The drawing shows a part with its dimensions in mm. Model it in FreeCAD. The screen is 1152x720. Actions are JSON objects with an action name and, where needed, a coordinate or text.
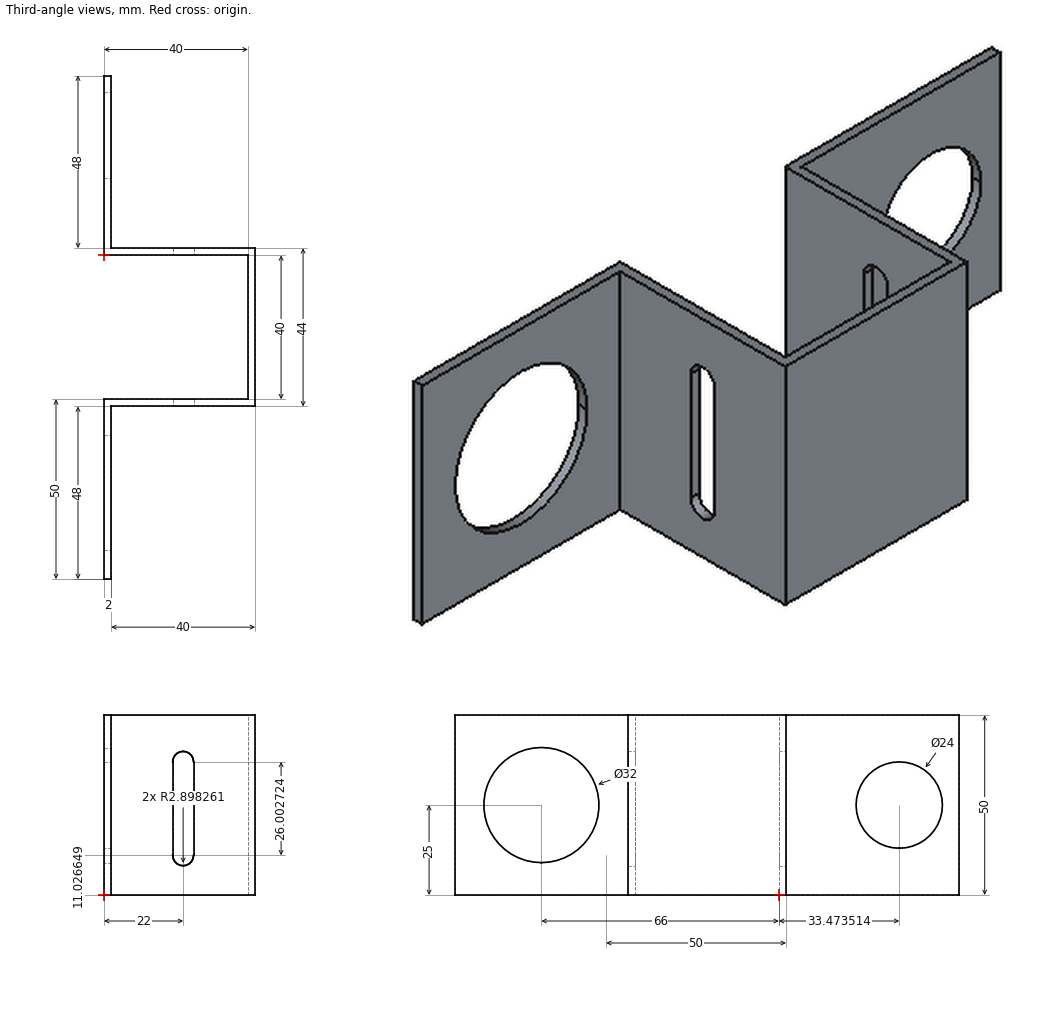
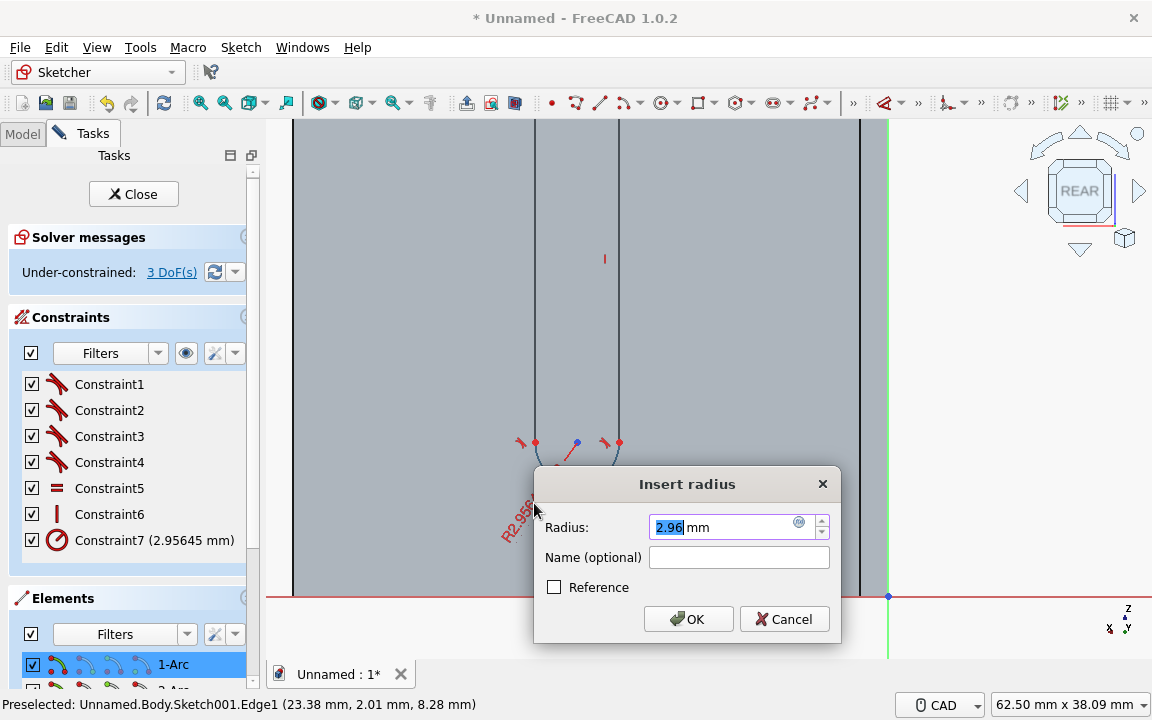
{"action": "type", "text": "2.898261"}
{"action": "key", "text": "Return"}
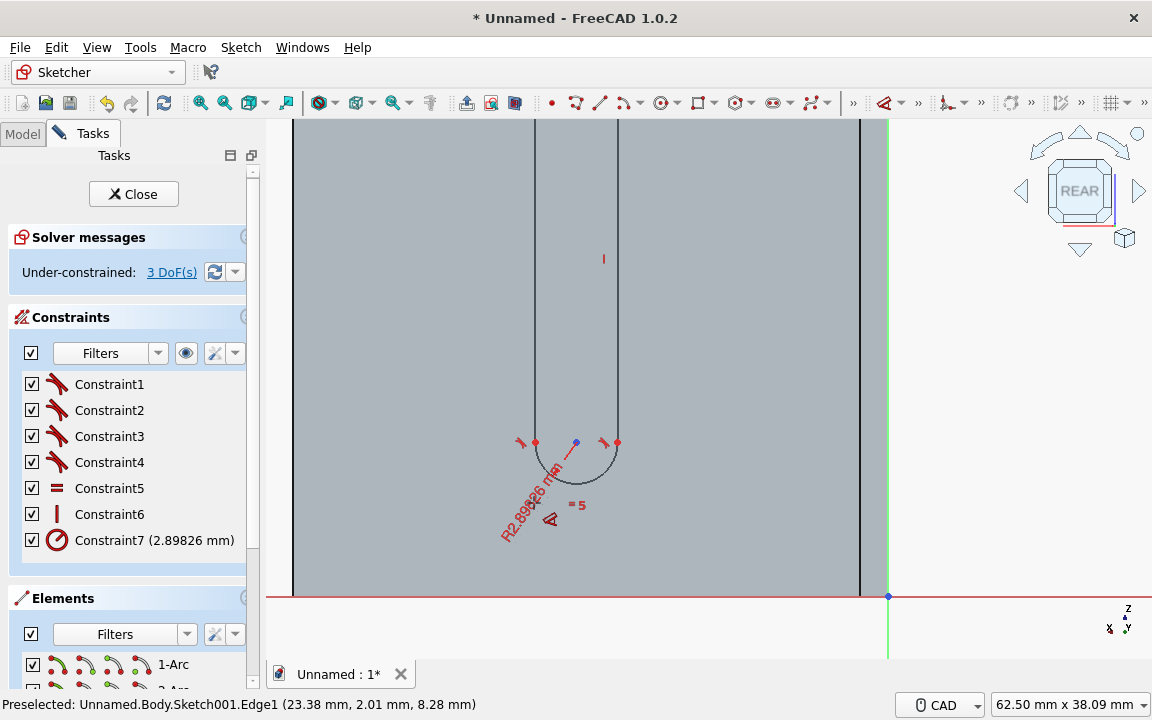
{"action": "left_click", "coordinate": [576, 443]}
{"action": "left_click", "coordinate": [732, 631]}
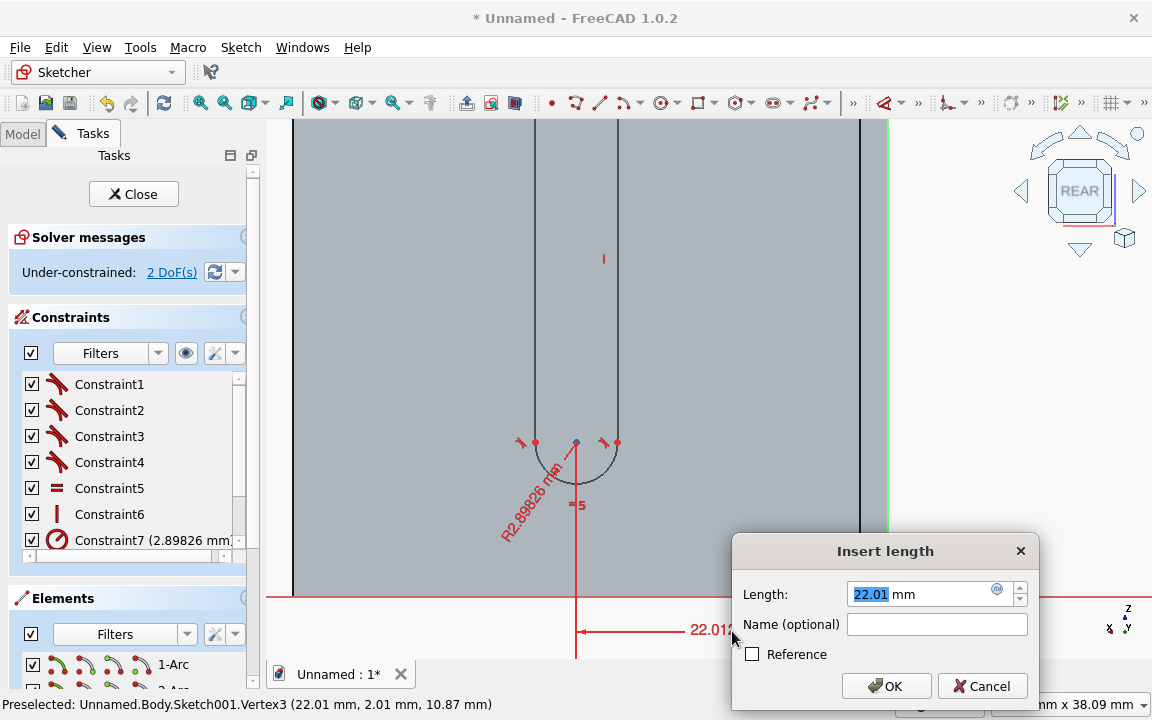
{"action": "type", "text": "22"}
{"action": "key", "text": "Return"}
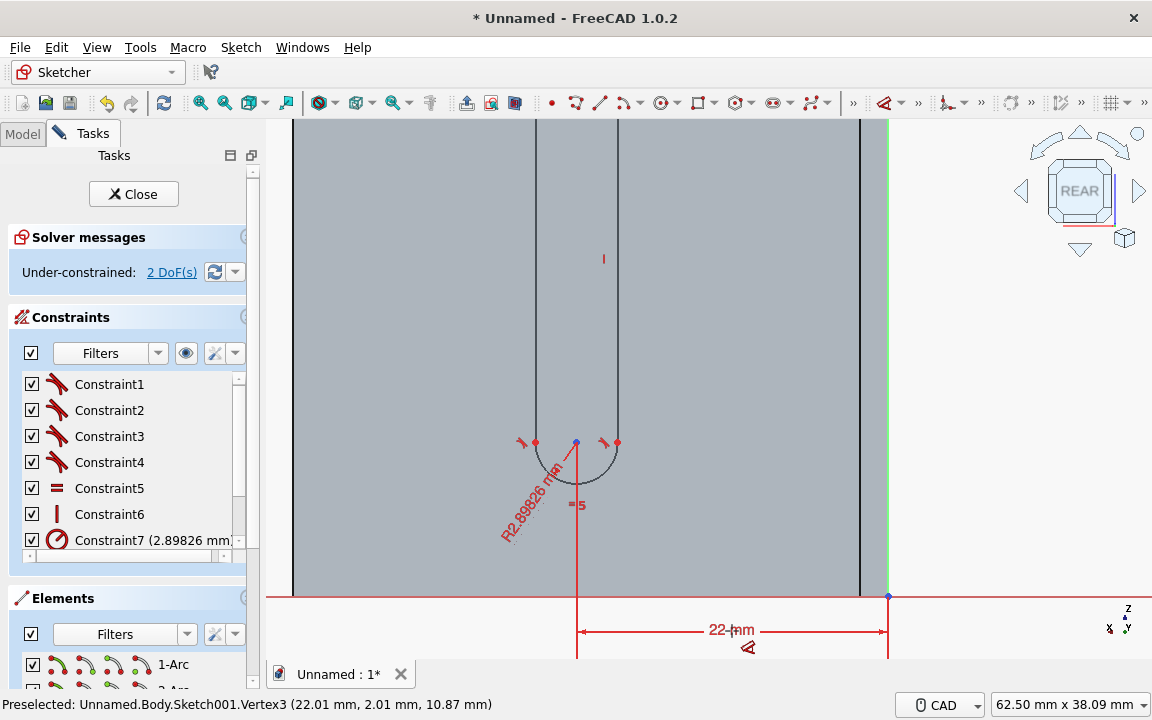
{"action": "left_click", "coordinate": [536, 332]}
{"action": "left_click", "coordinate": [502, 295]}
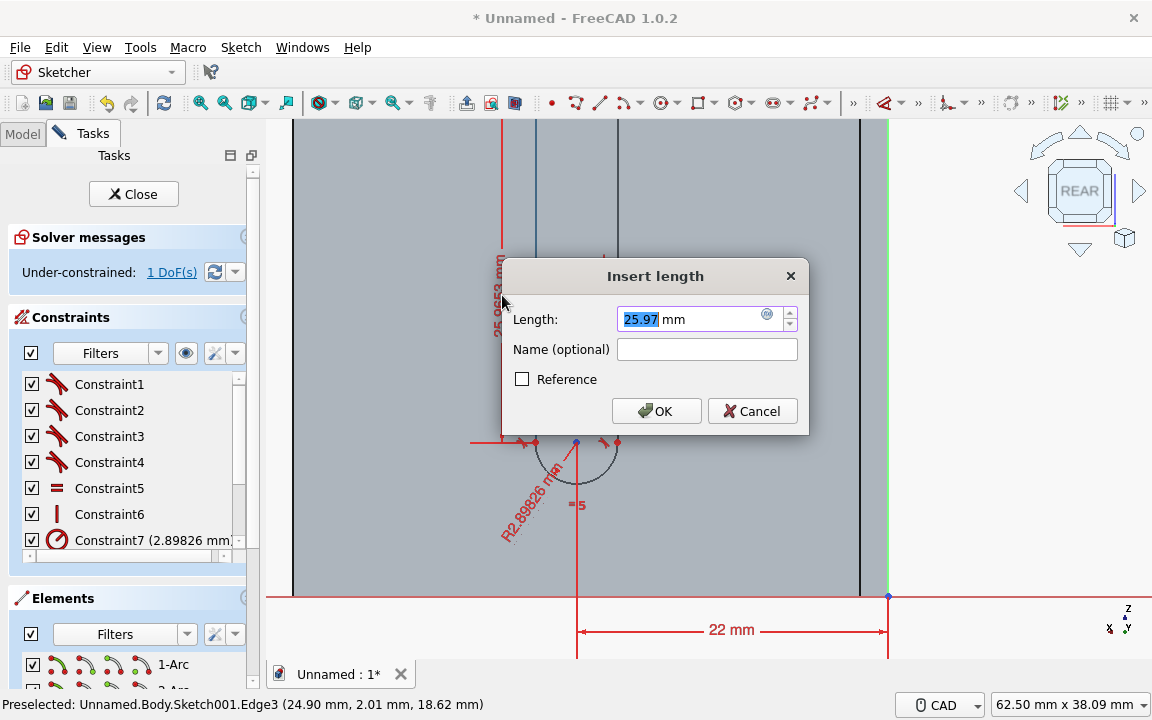
{"action": "type", "text": "26.002724"}
{"action": "key", "text": "Return"}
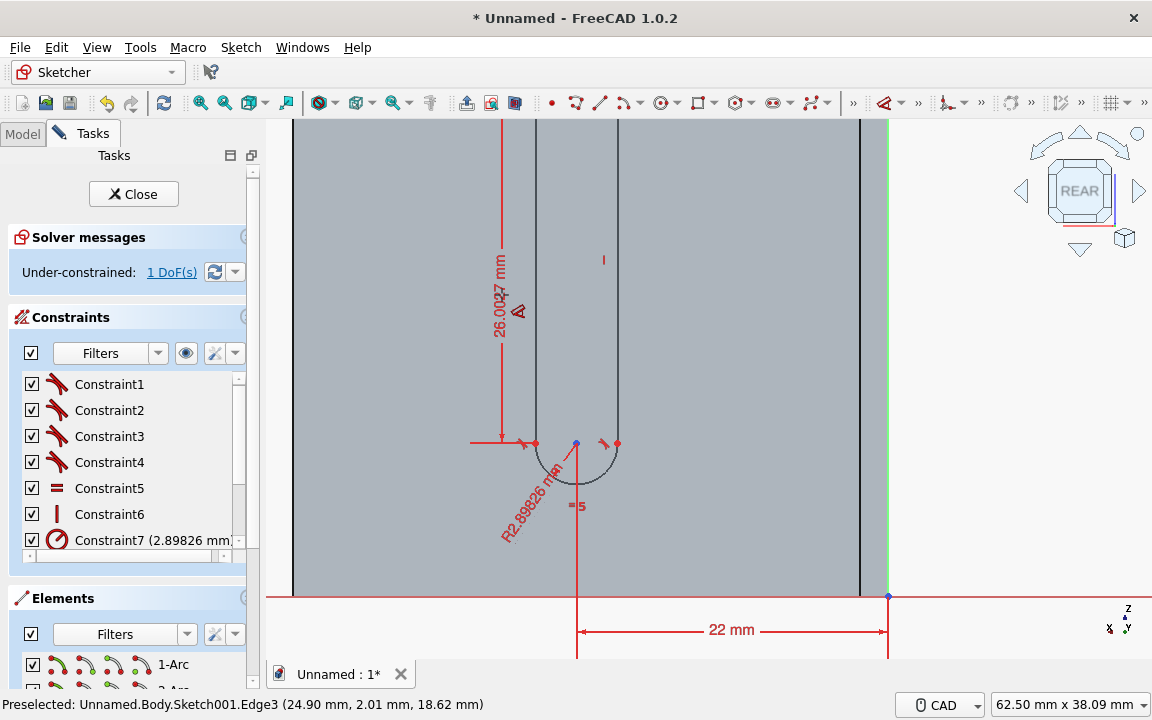
{"action": "left_click", "coordinate": [536, 443]}
{"action": "left_click", "coordinate": [922, 520]}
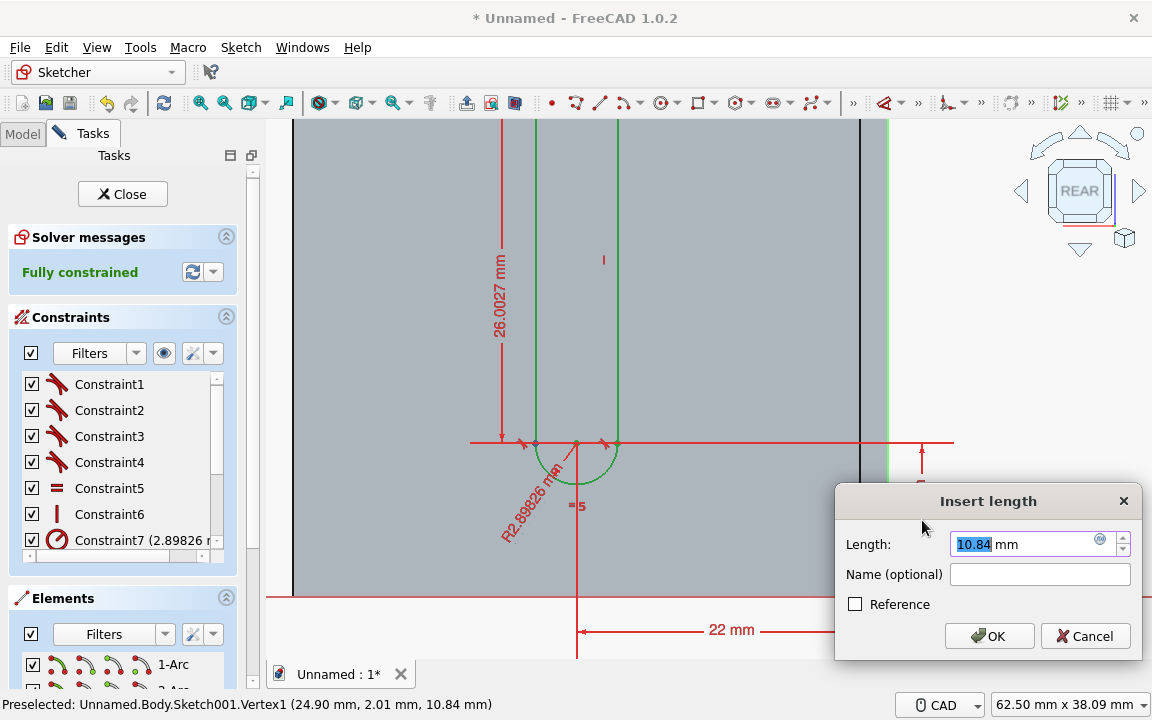
{"action": "type", "text": "11.026649"}
{"action": "key", "text": "Return"}
{"action": "key", "text": "Escape"}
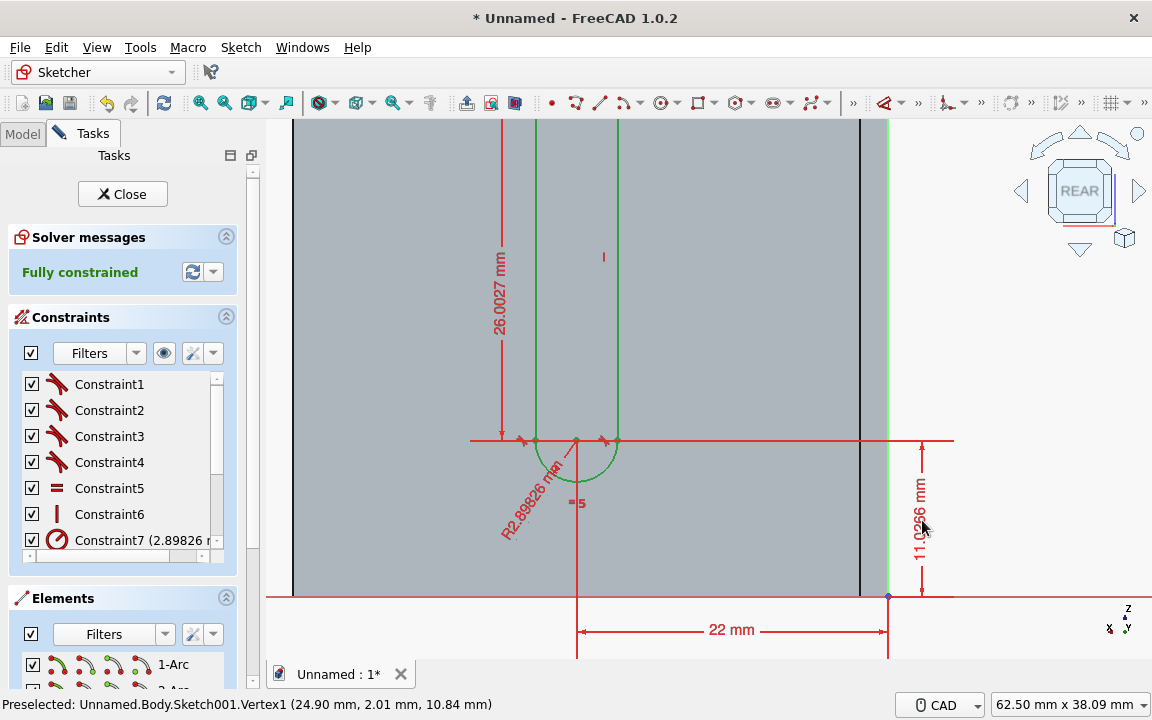
{"action": "left_click", "coordinate": [123, 194]}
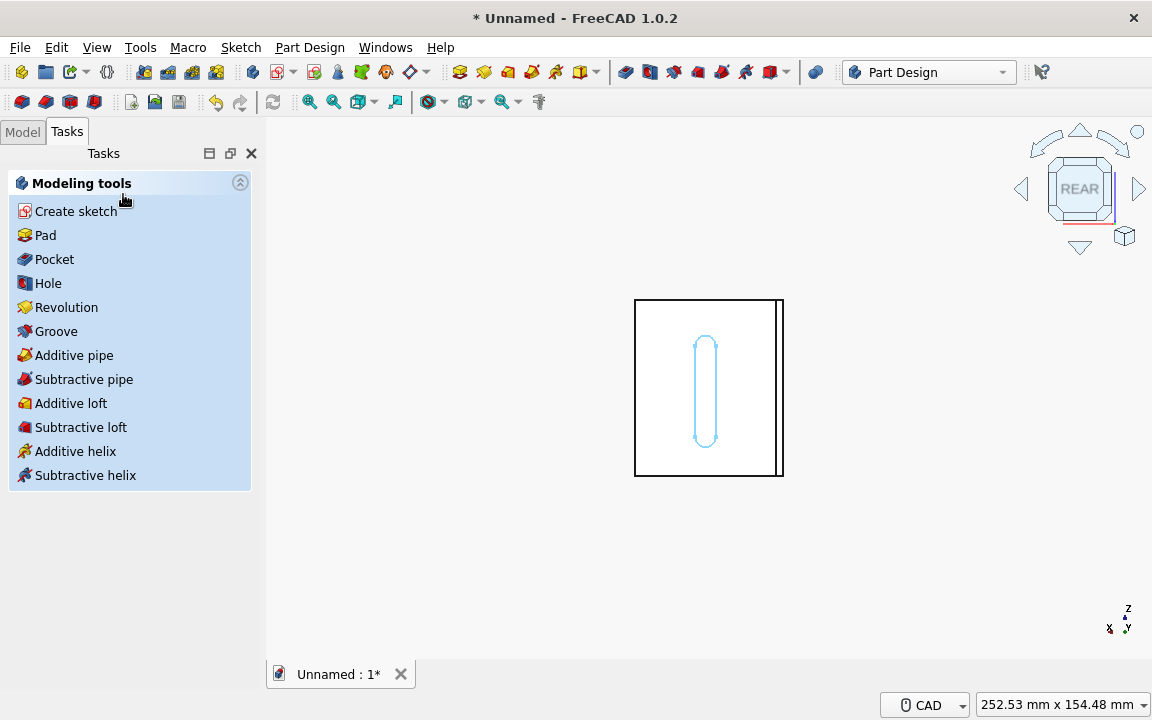
{"action": "left_click", "coordinate": [626, 72]}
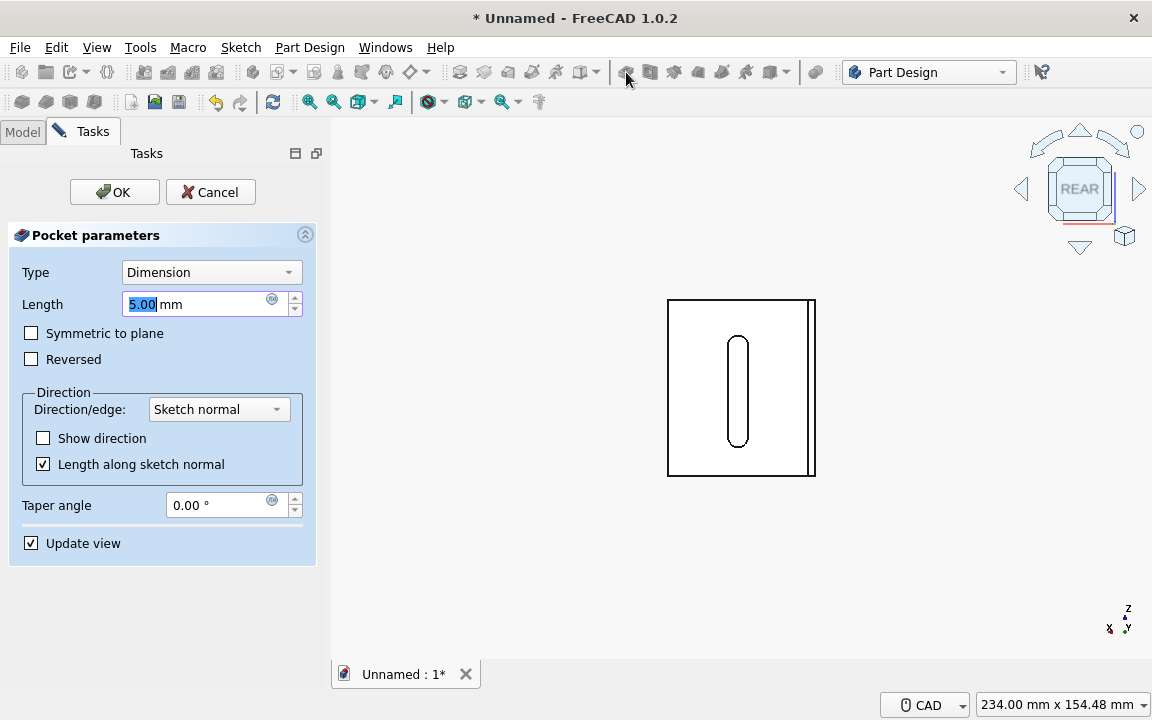
{"action": "type", "text": "50"}
{"action": "key", "text": "Tab"}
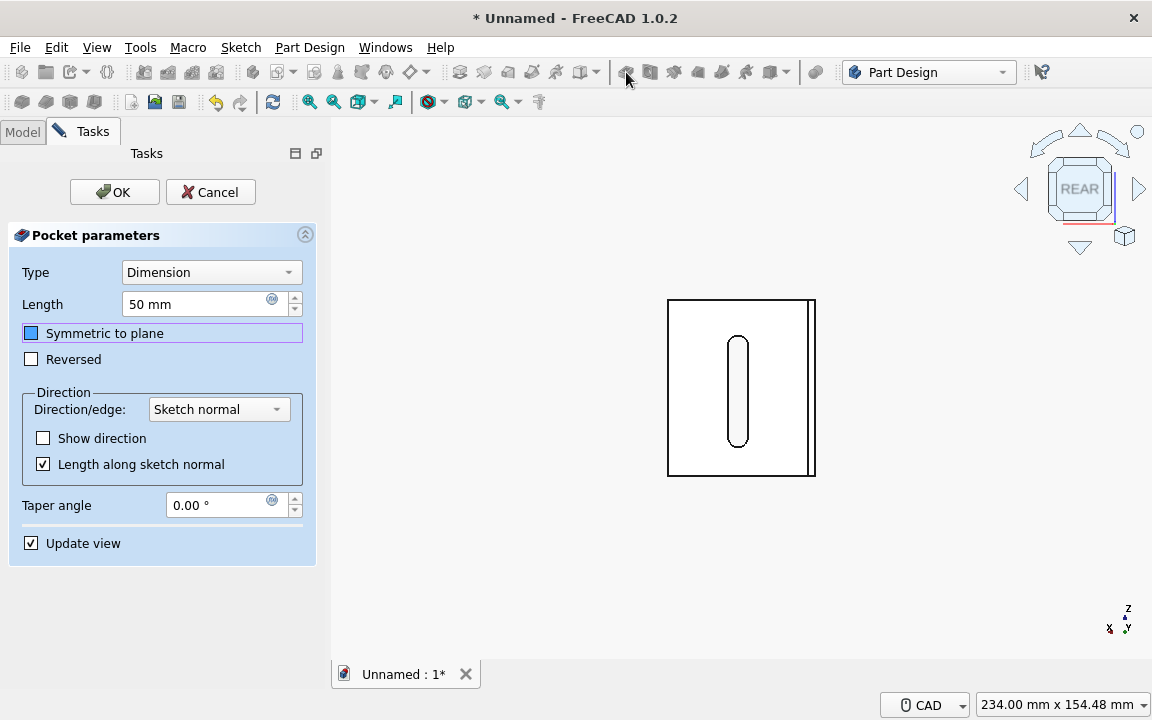
{"action": "left_click", "coordinate": [115, 192]}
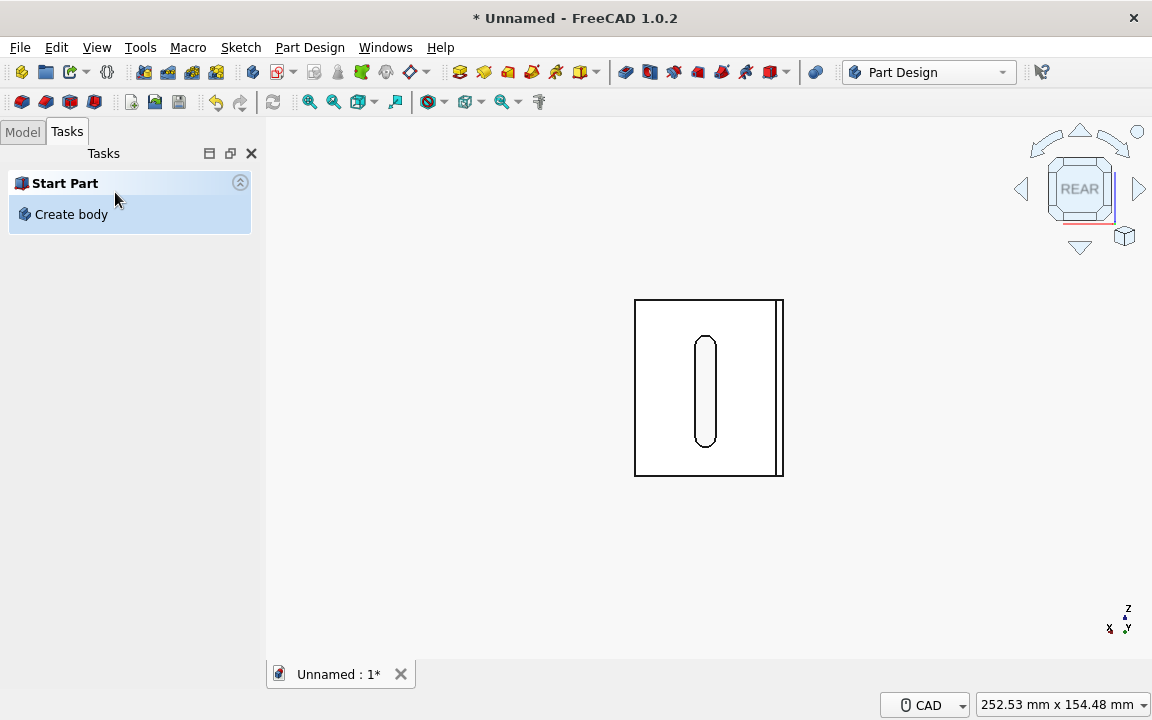
{"action": "left_click", "coordinate": [310, 102]}